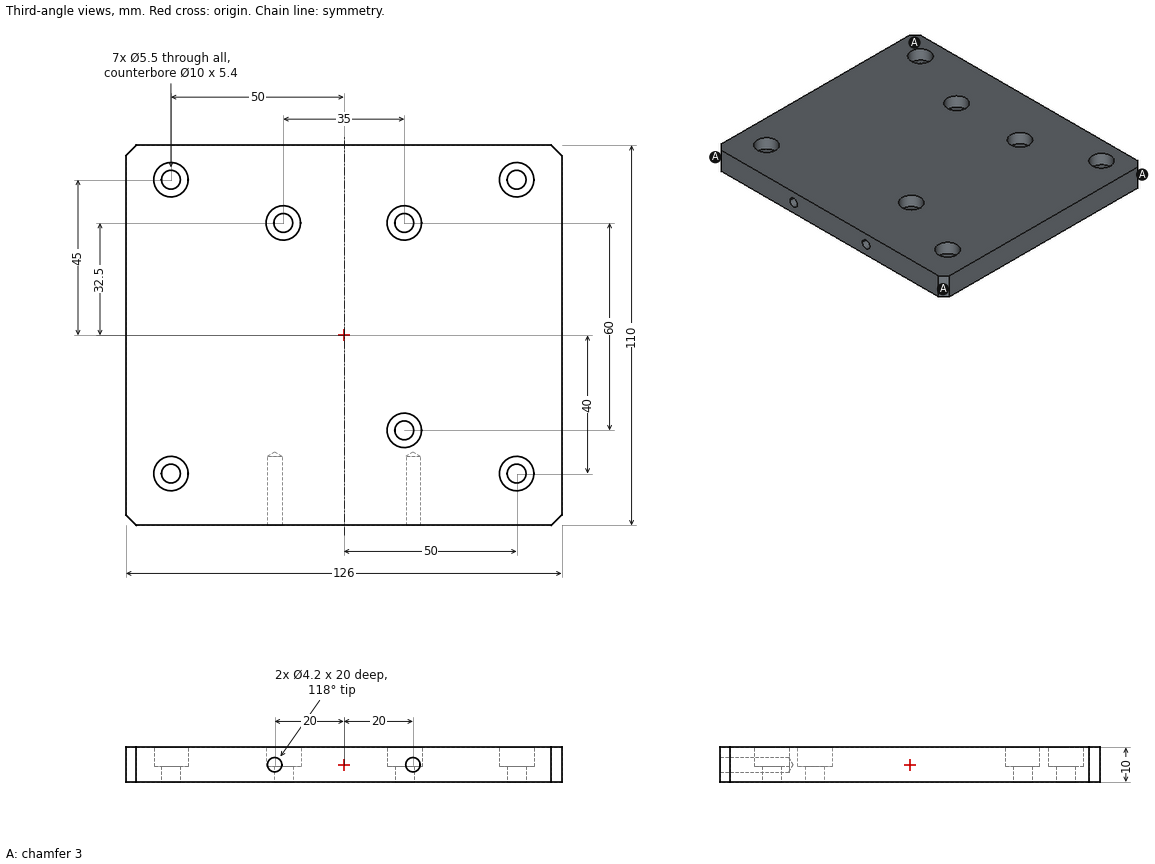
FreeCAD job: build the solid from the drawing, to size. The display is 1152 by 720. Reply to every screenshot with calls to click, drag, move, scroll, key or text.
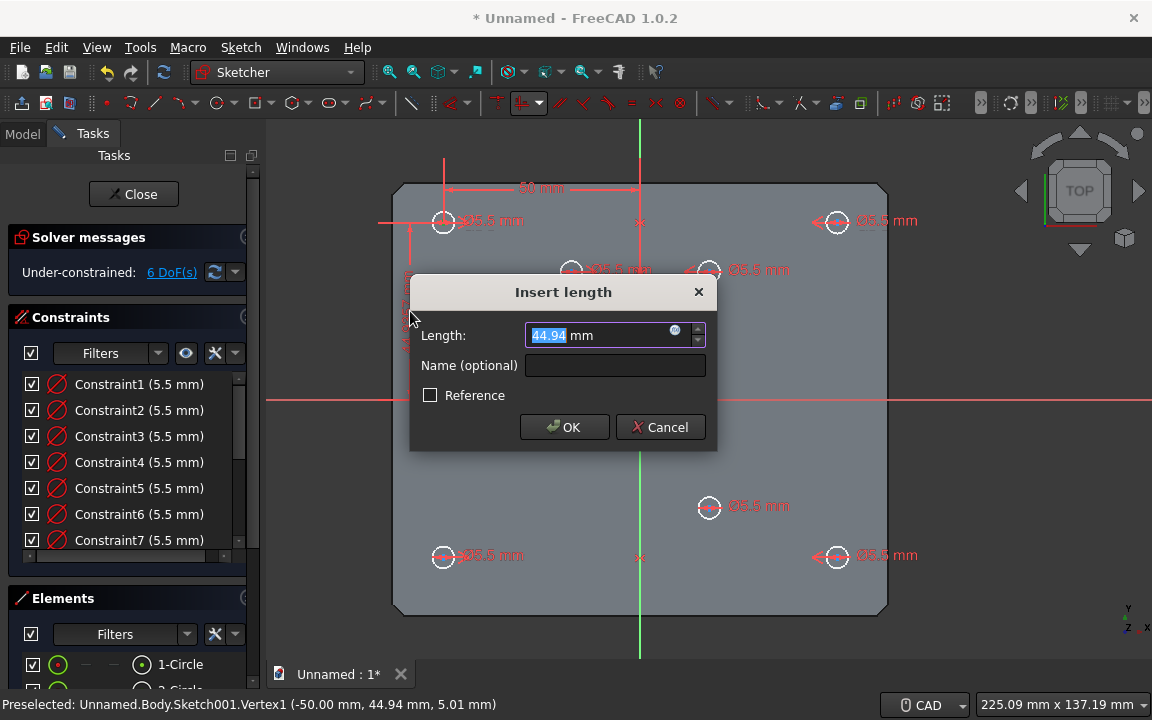
text(45)
key(Return)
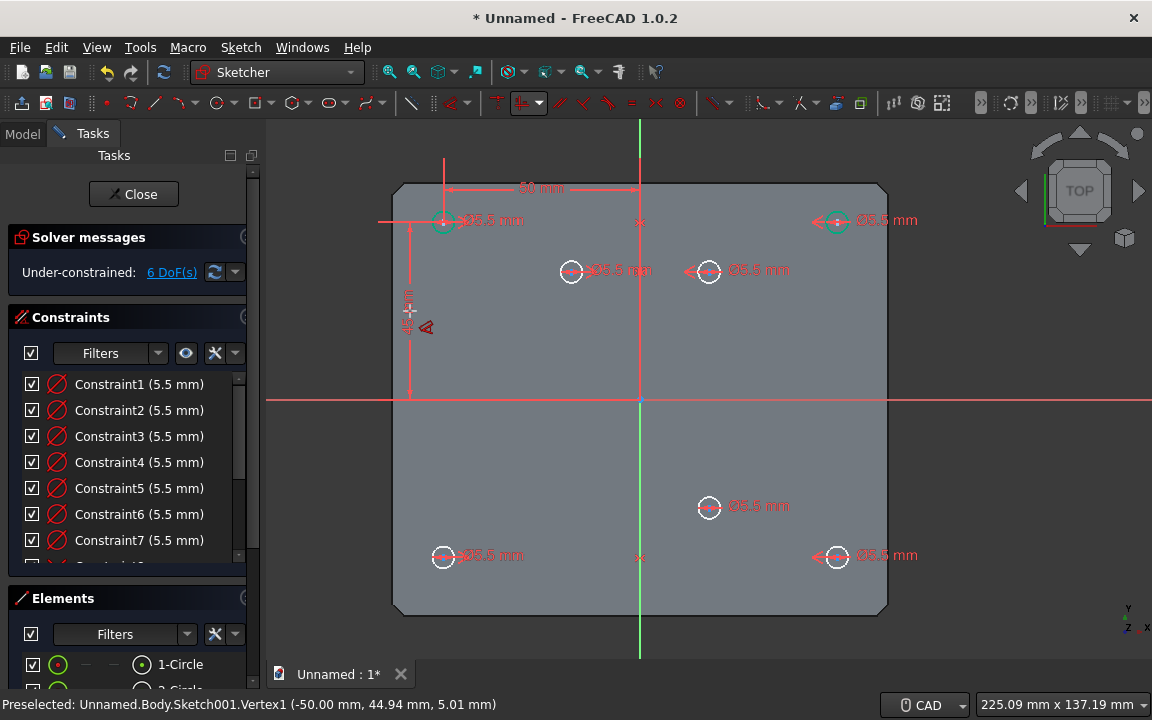
click(837, 557)
click(739, 591)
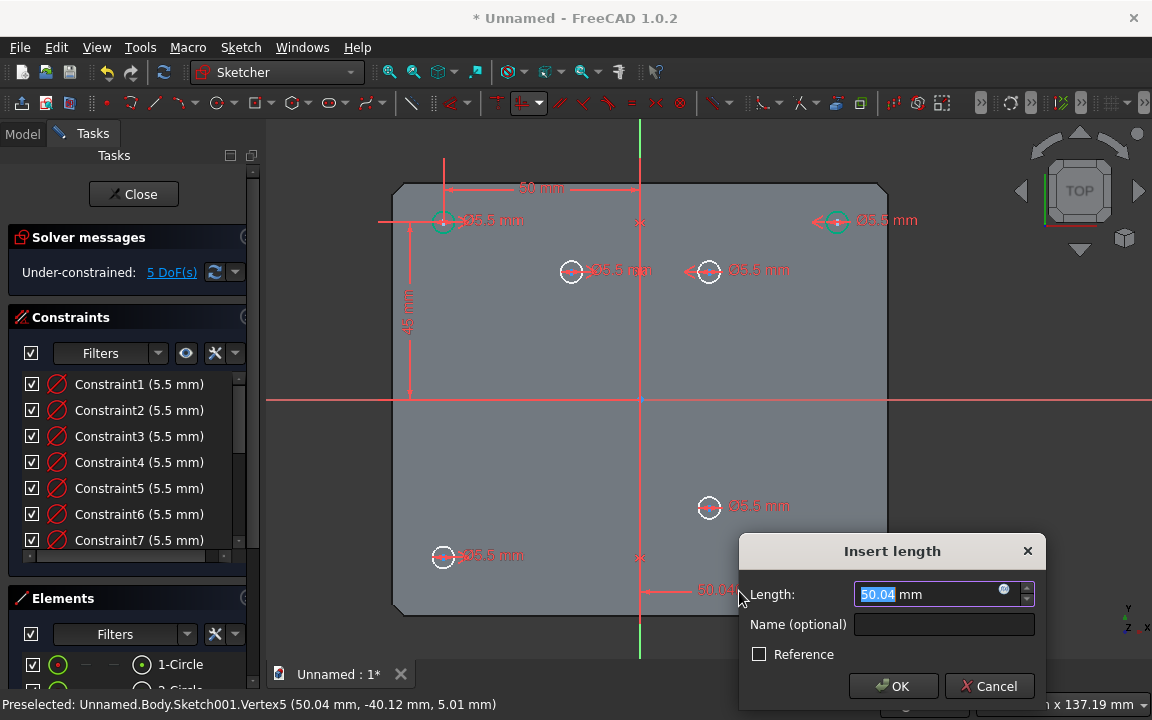
text(50)
key(Return)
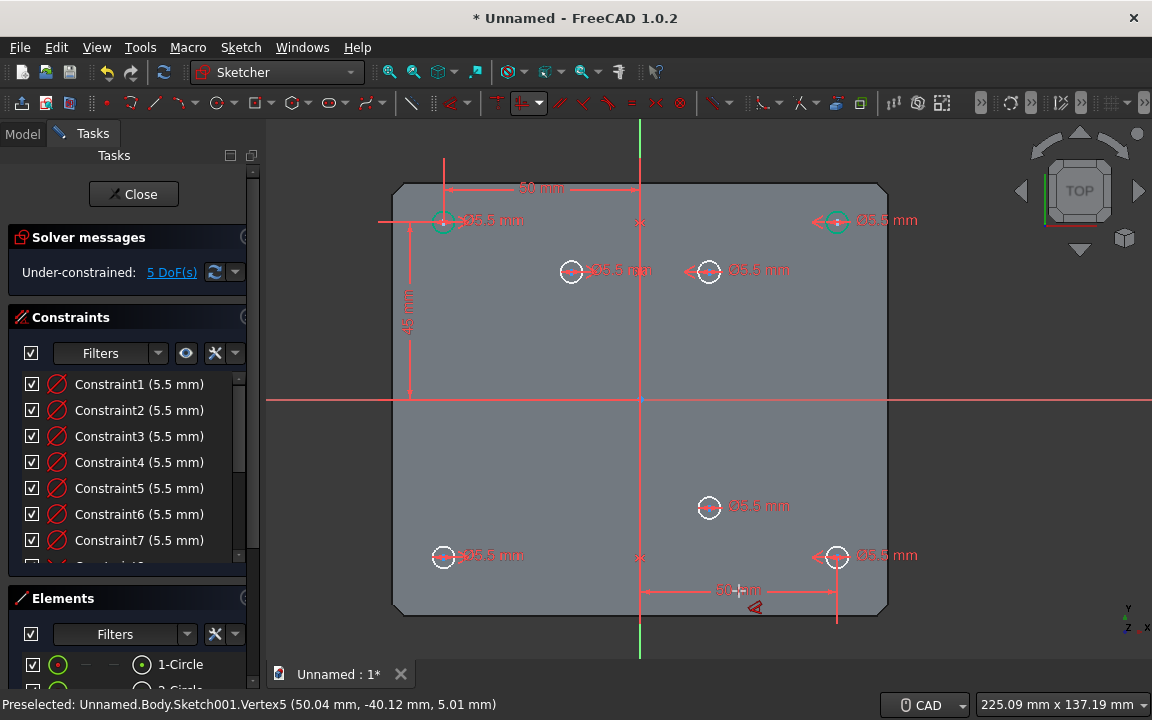
click(837, 557)
click(871, 478)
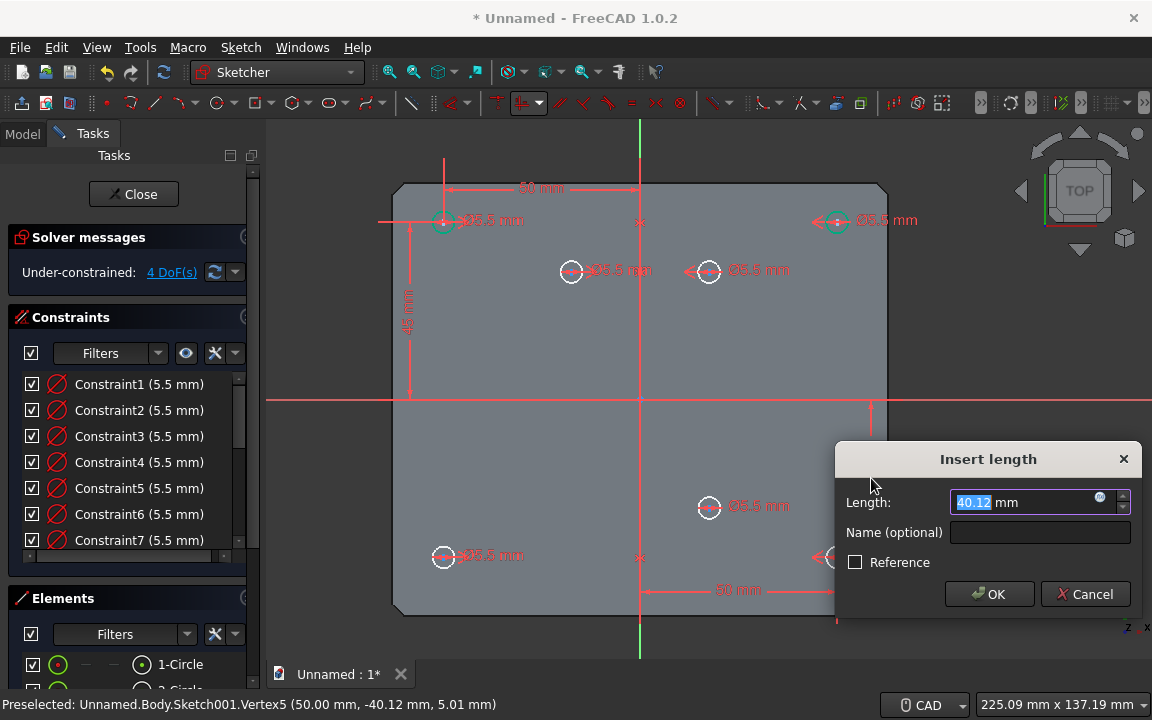
text(40)
key(Return)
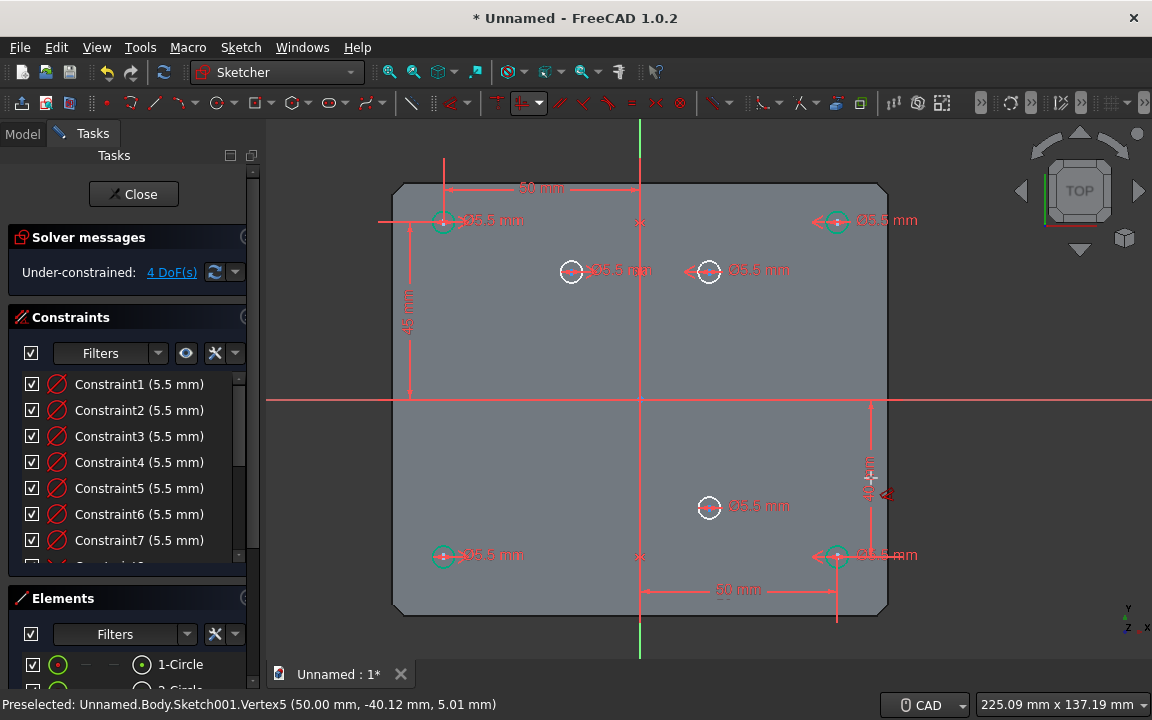
click(572, 272)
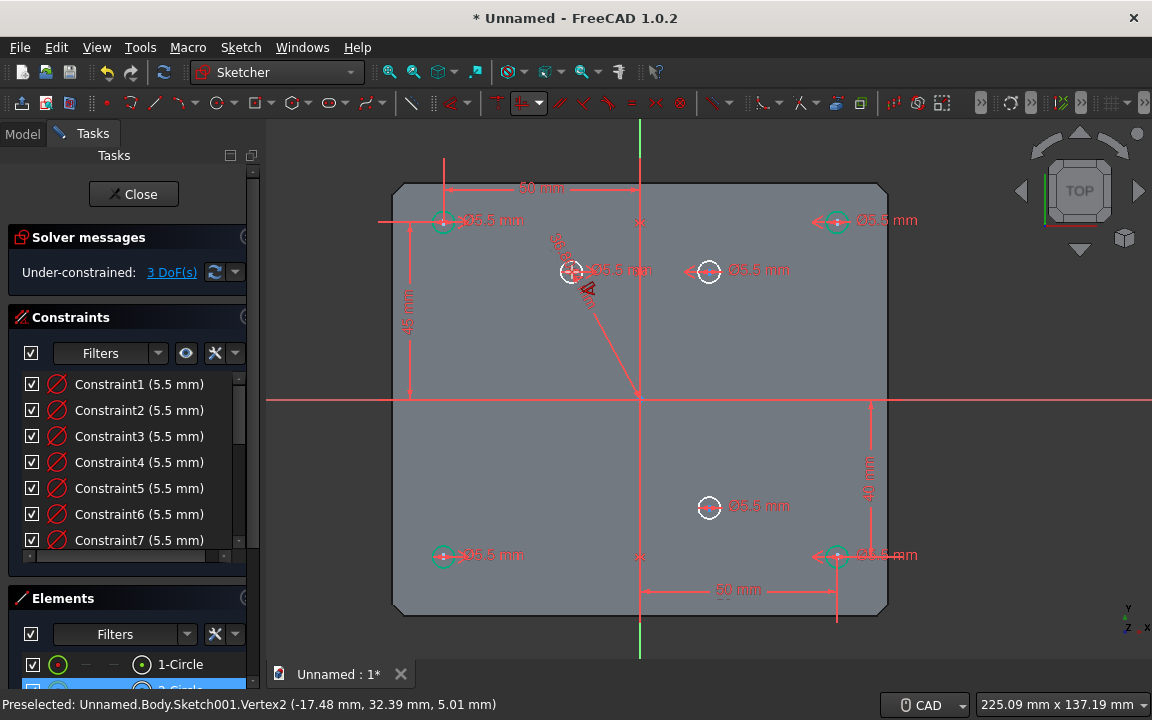
click(709, 272)
click(609, 238)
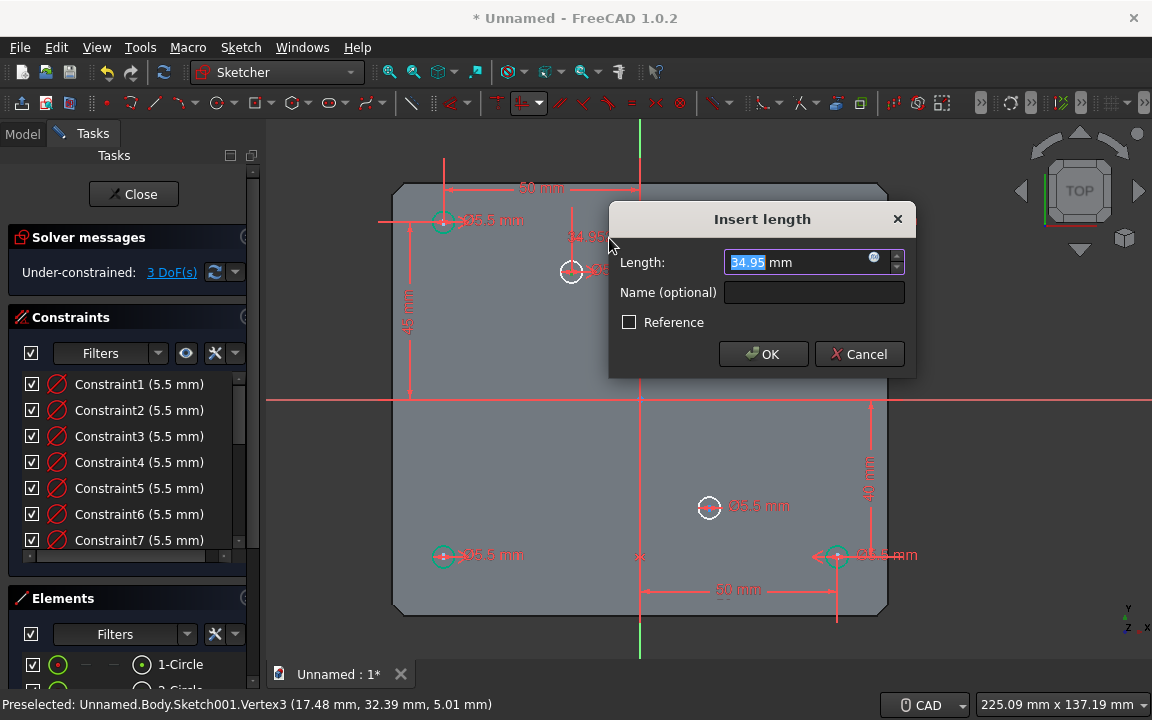
text(35)
key(Return)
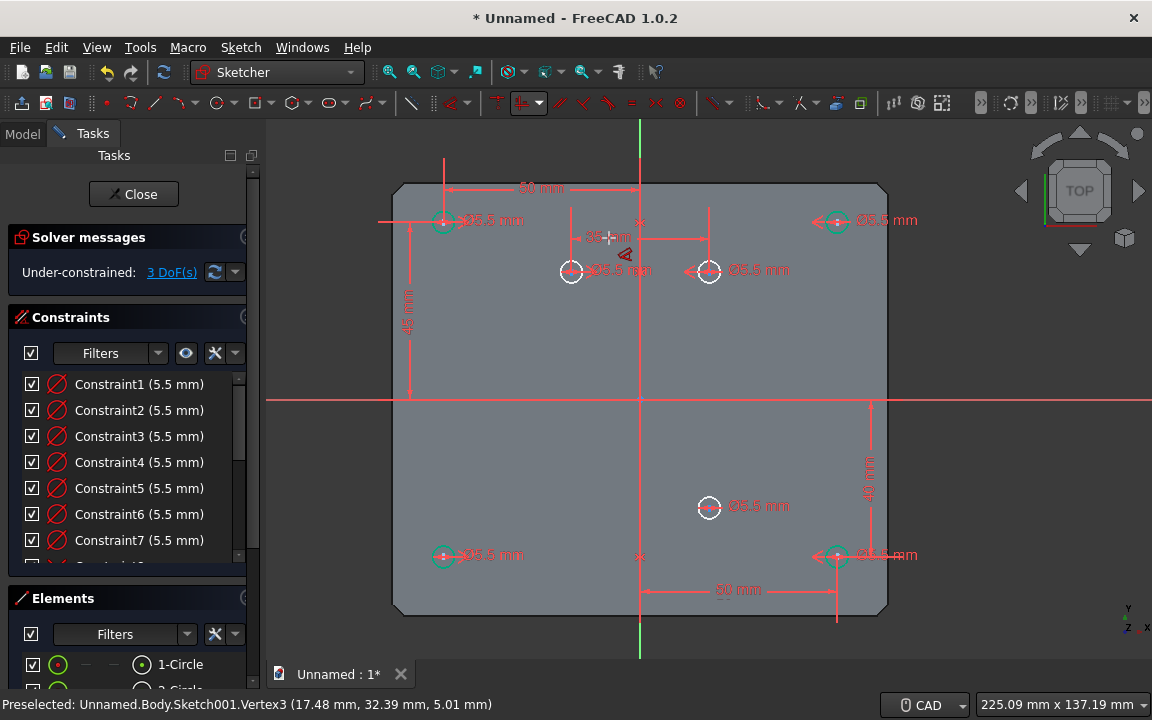
click(571, 272)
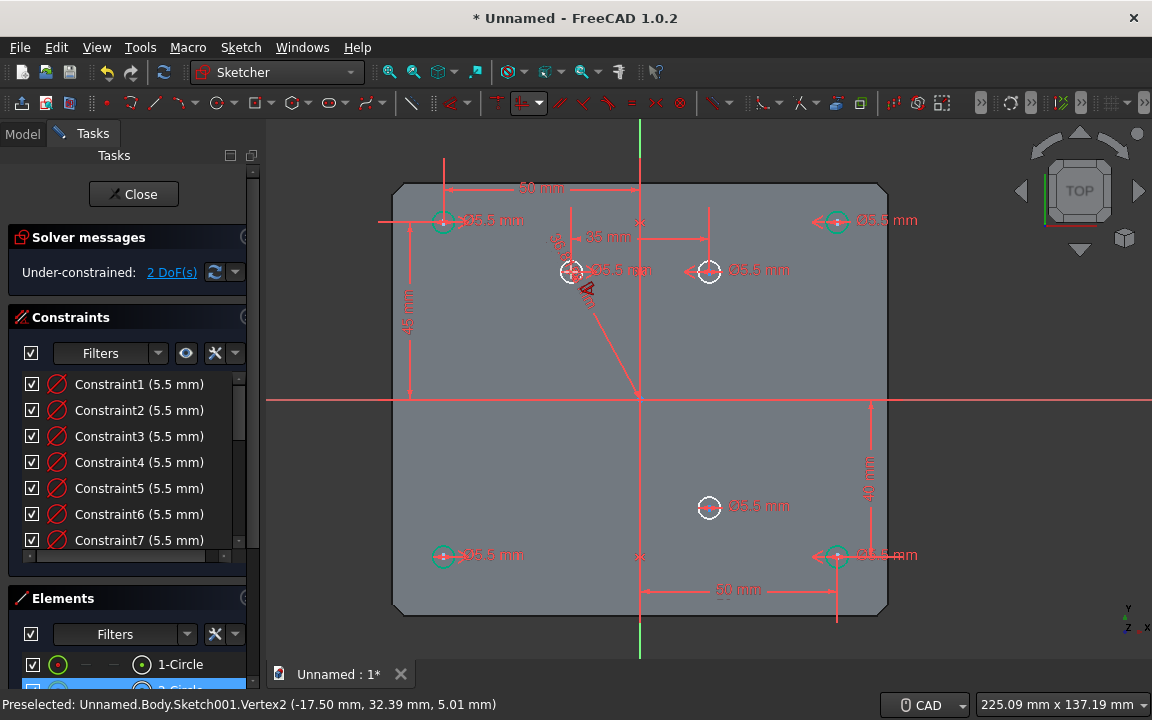
click(709, 508)
click(609, 542)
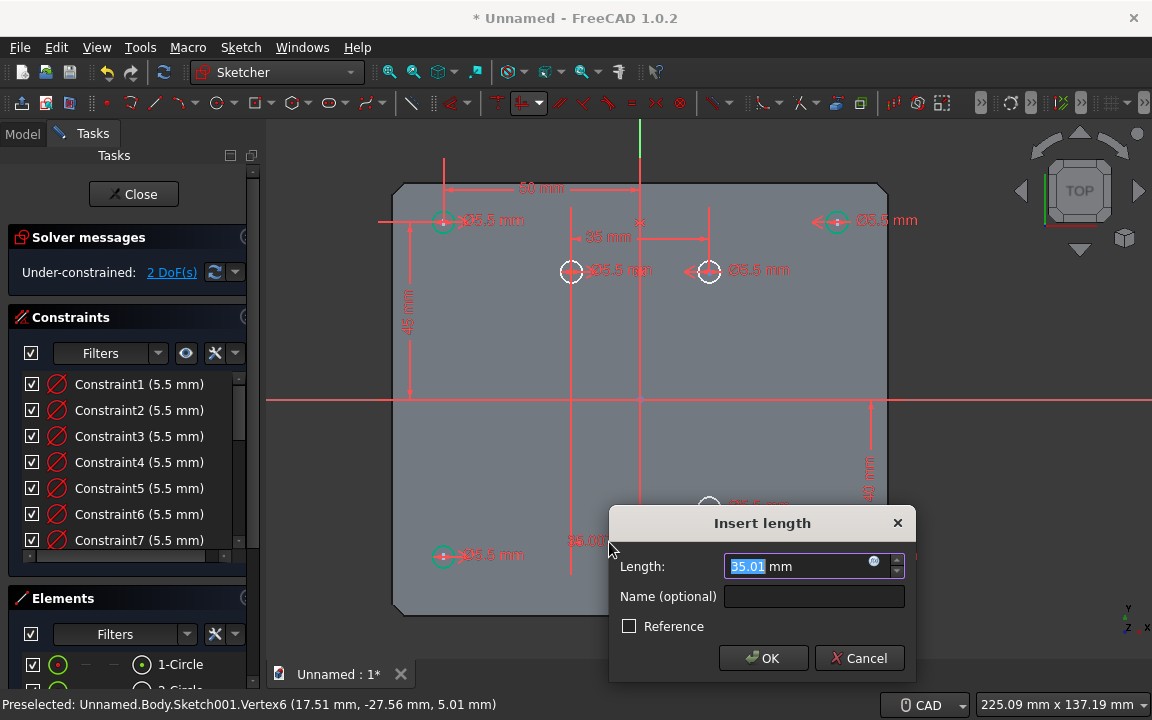
text(35)
key(Return)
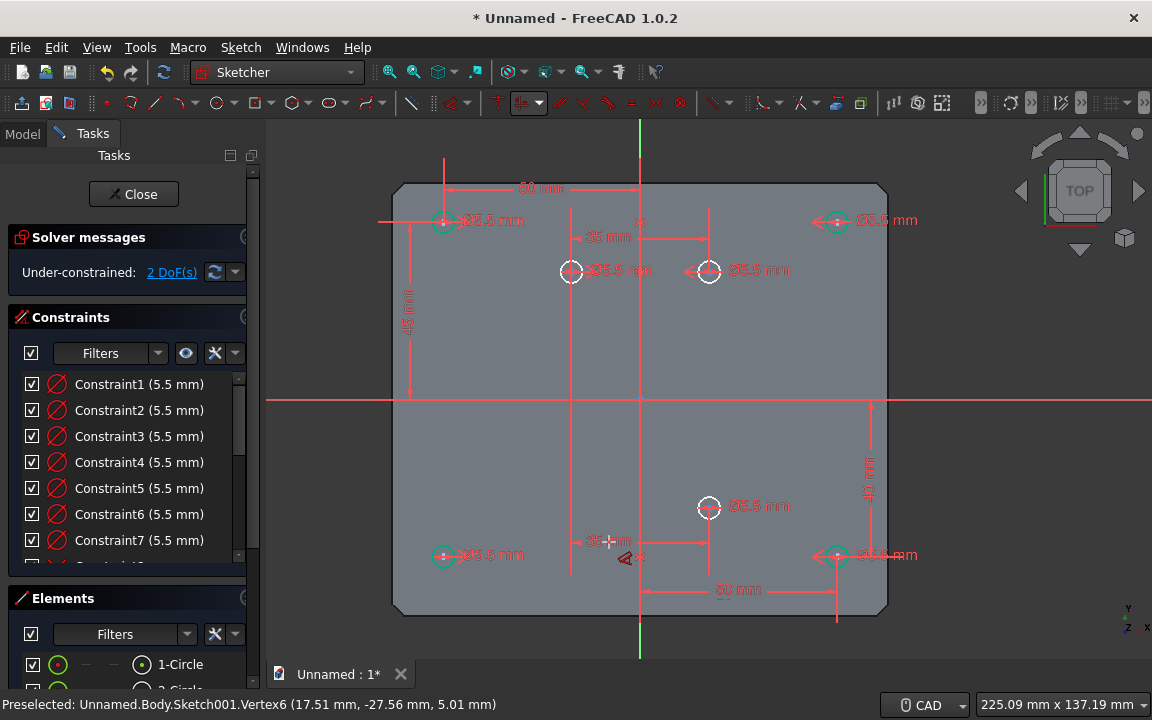
click(709, 272)